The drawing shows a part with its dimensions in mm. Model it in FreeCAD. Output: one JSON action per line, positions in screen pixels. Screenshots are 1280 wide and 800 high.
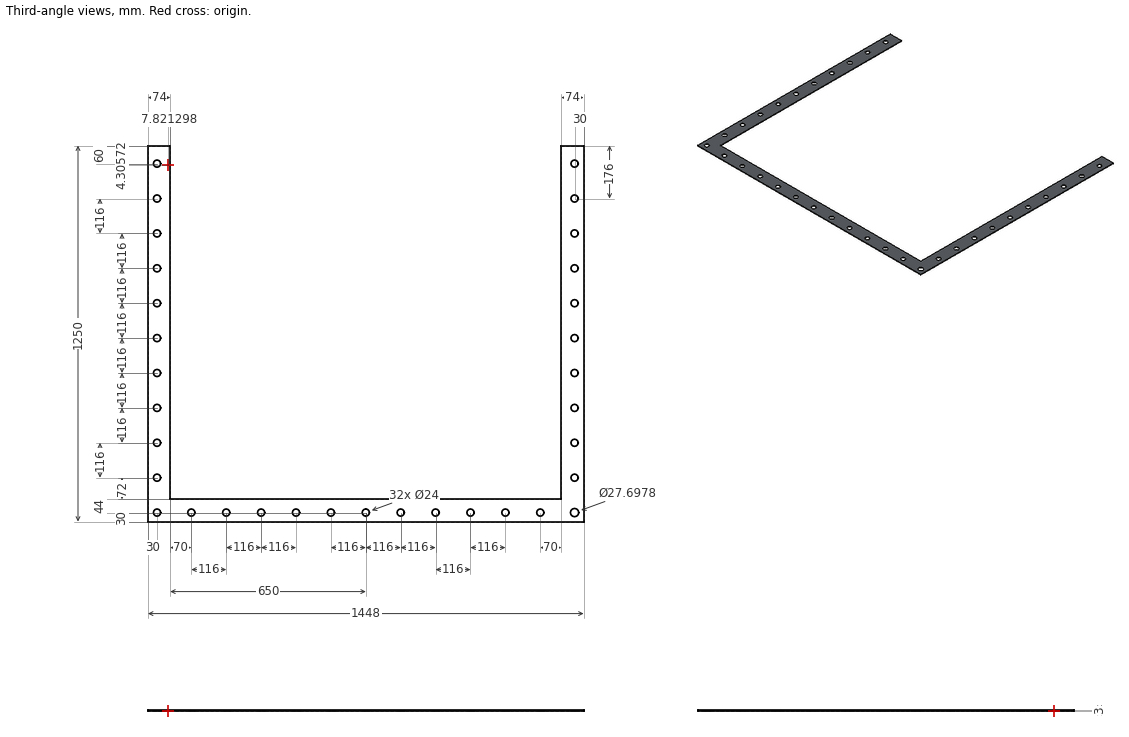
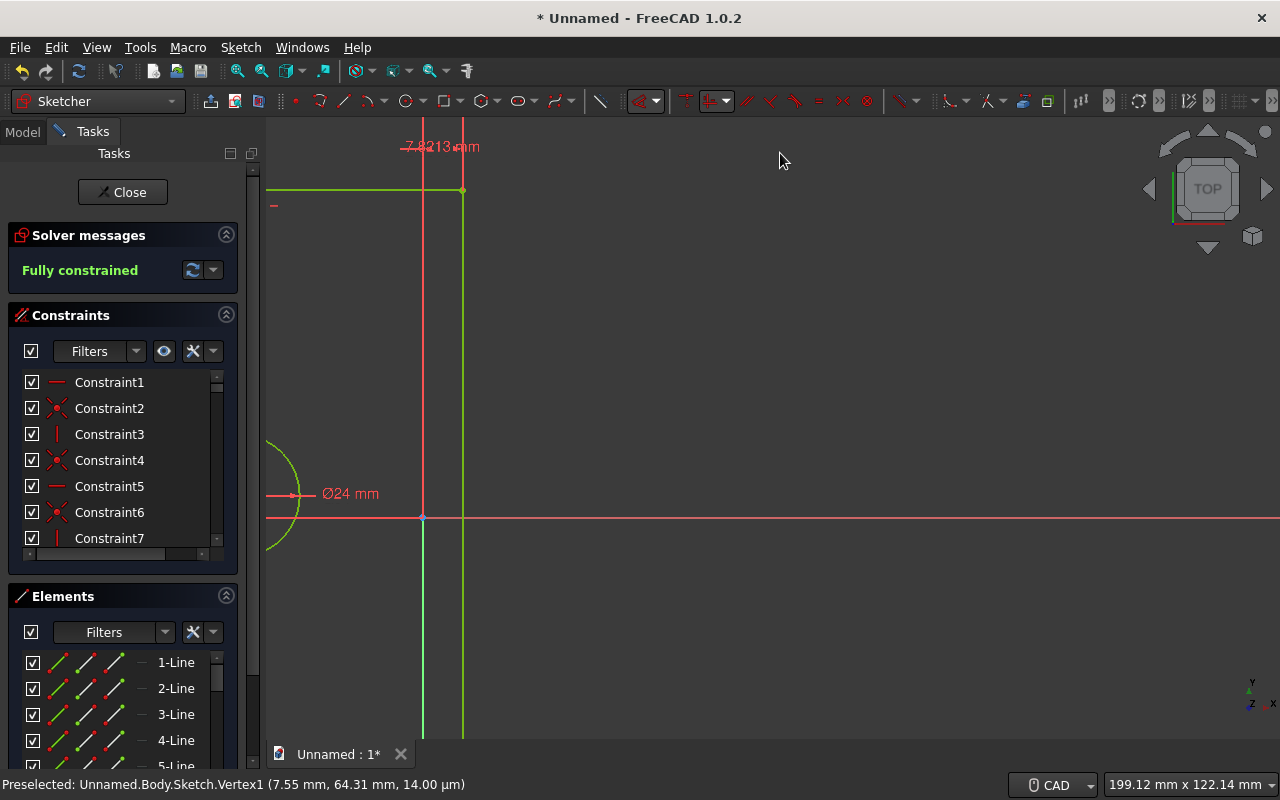
{"action": "left_click", "coordinate": [123, 192]}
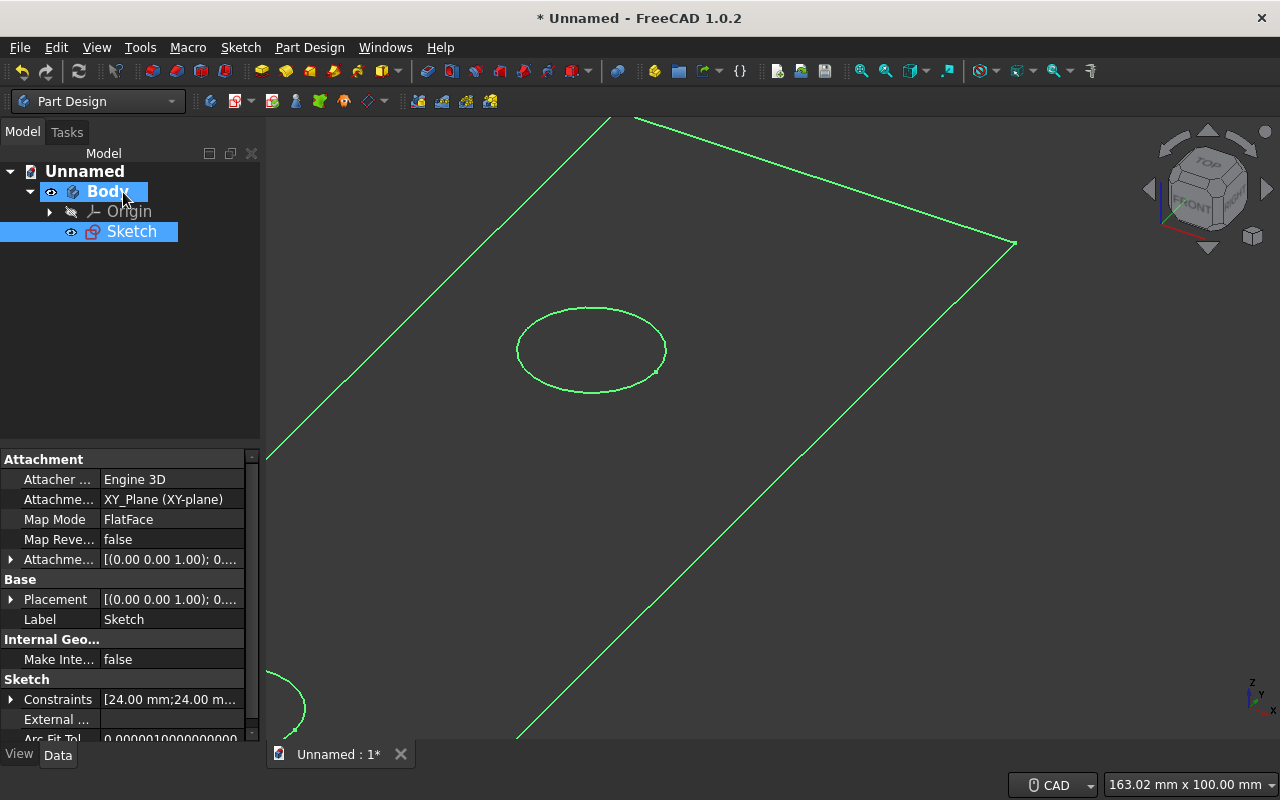
{"action": "left_click", "coordinate": [262, 72]}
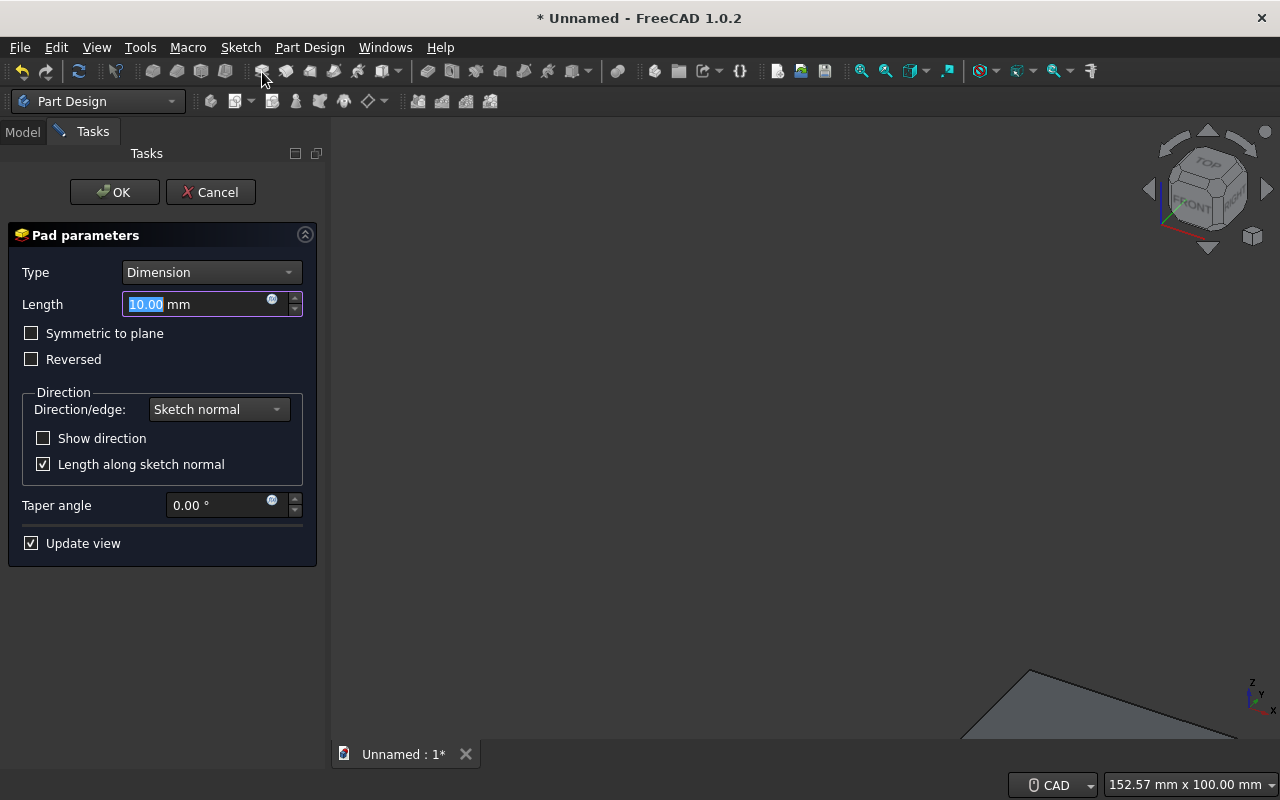
{"action": "type", "text": "3"}
{"action": "key", "text": "Tab"}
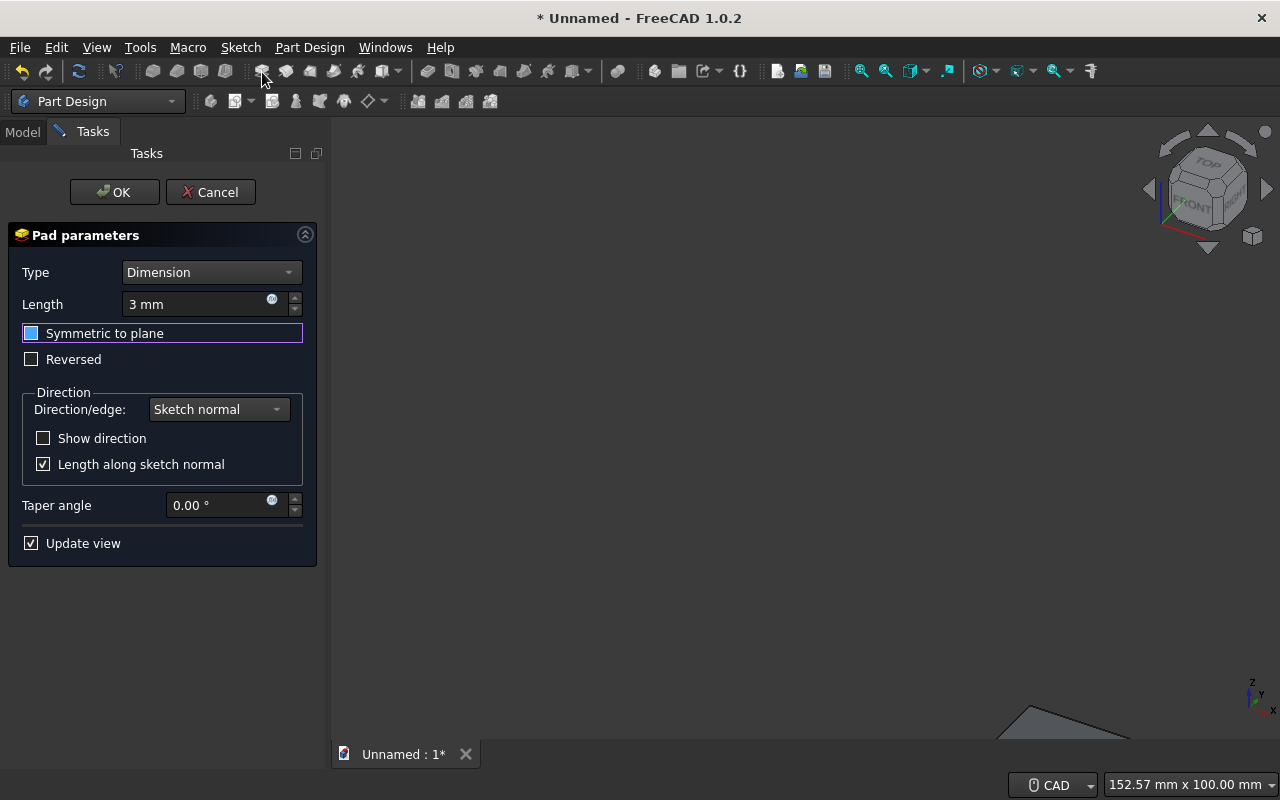
{"action": "left_click", "coordinate": [115, 192]}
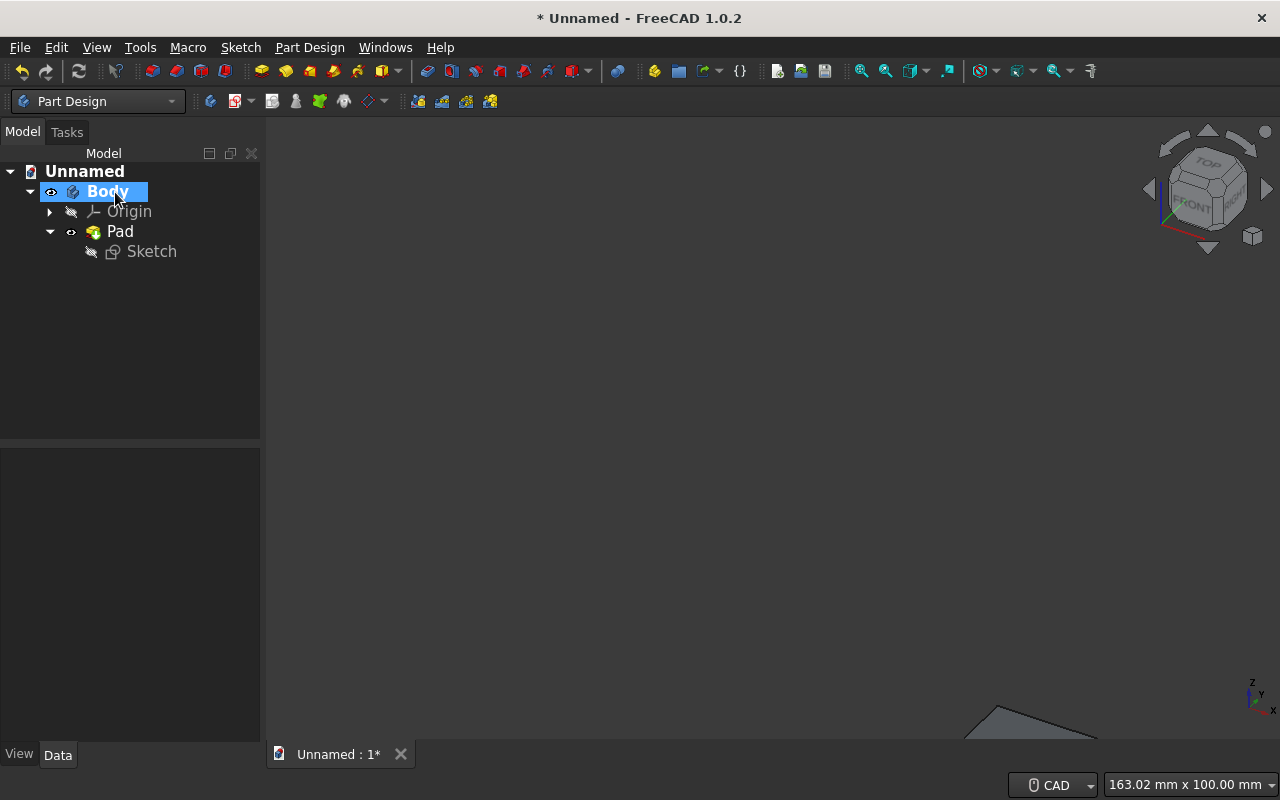
{"action": "key", "text": "0"}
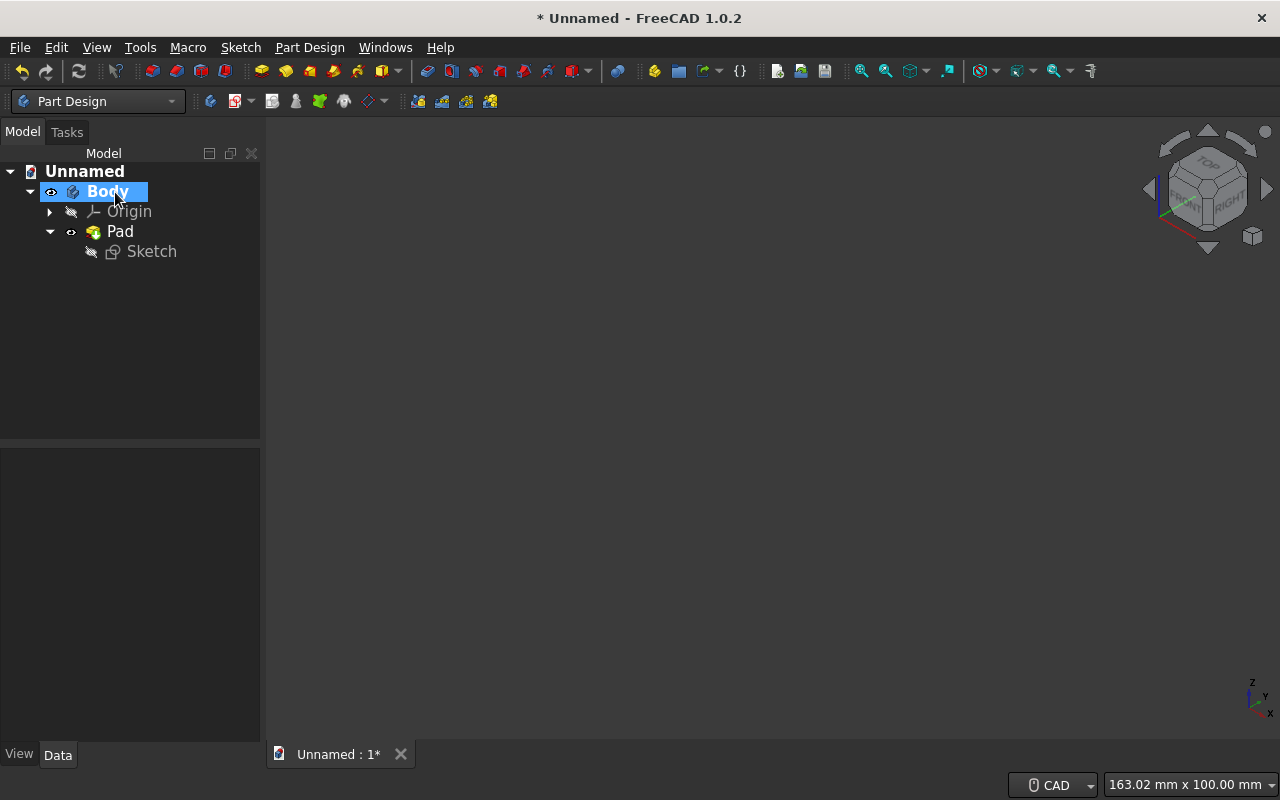
{"action": "left_click", "coordinate": [862, 72]}